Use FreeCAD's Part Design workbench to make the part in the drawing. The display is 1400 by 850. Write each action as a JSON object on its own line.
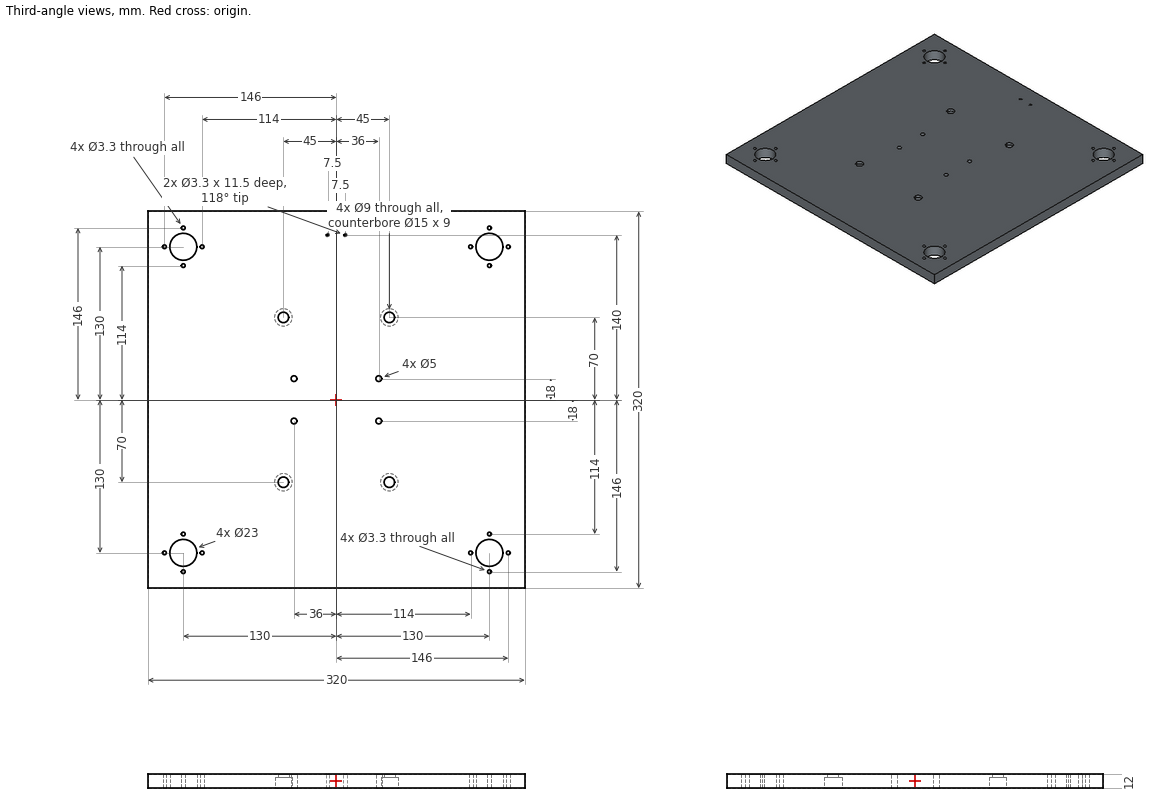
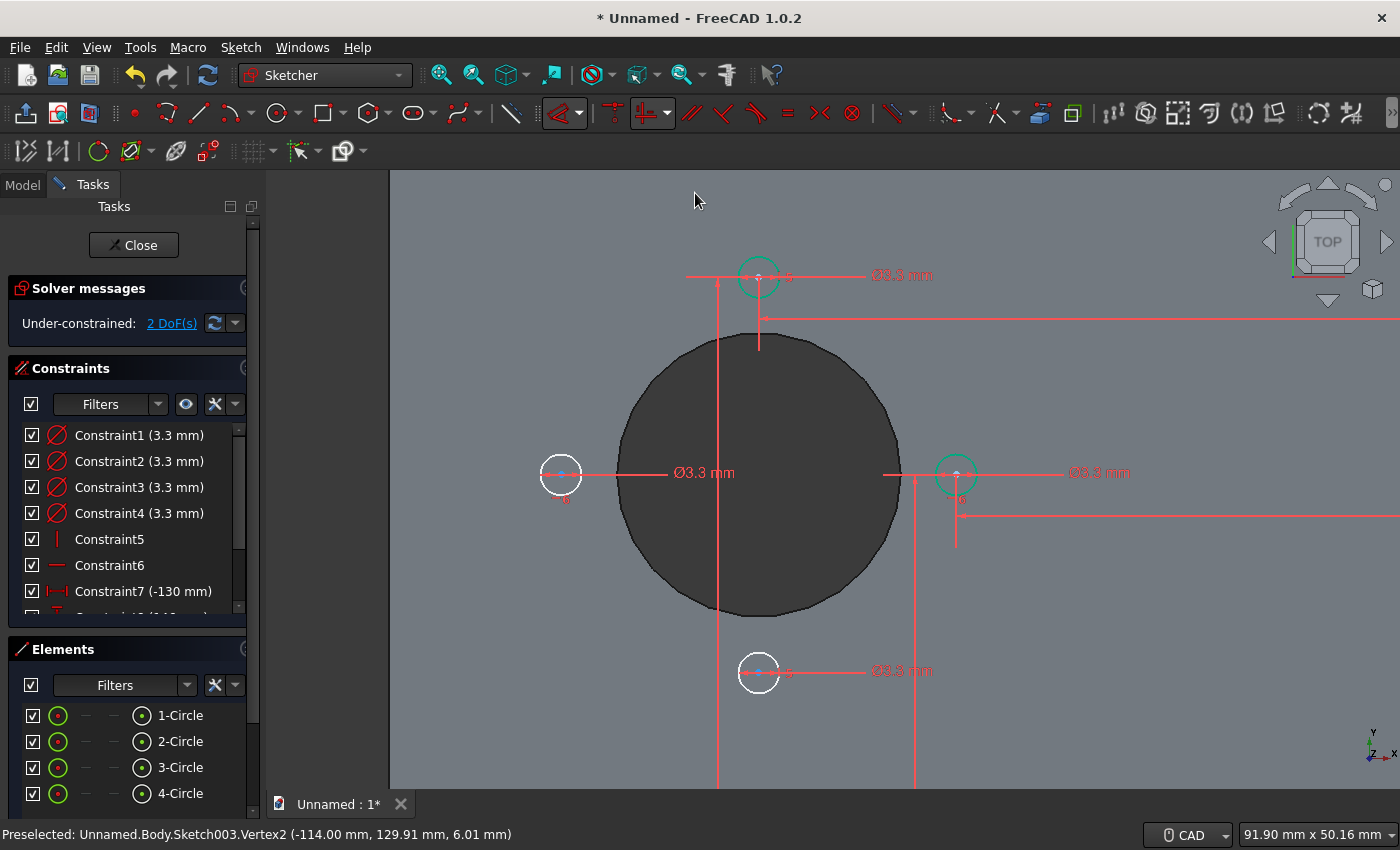
{"action": "left_click", "coordinate": [759, 673]}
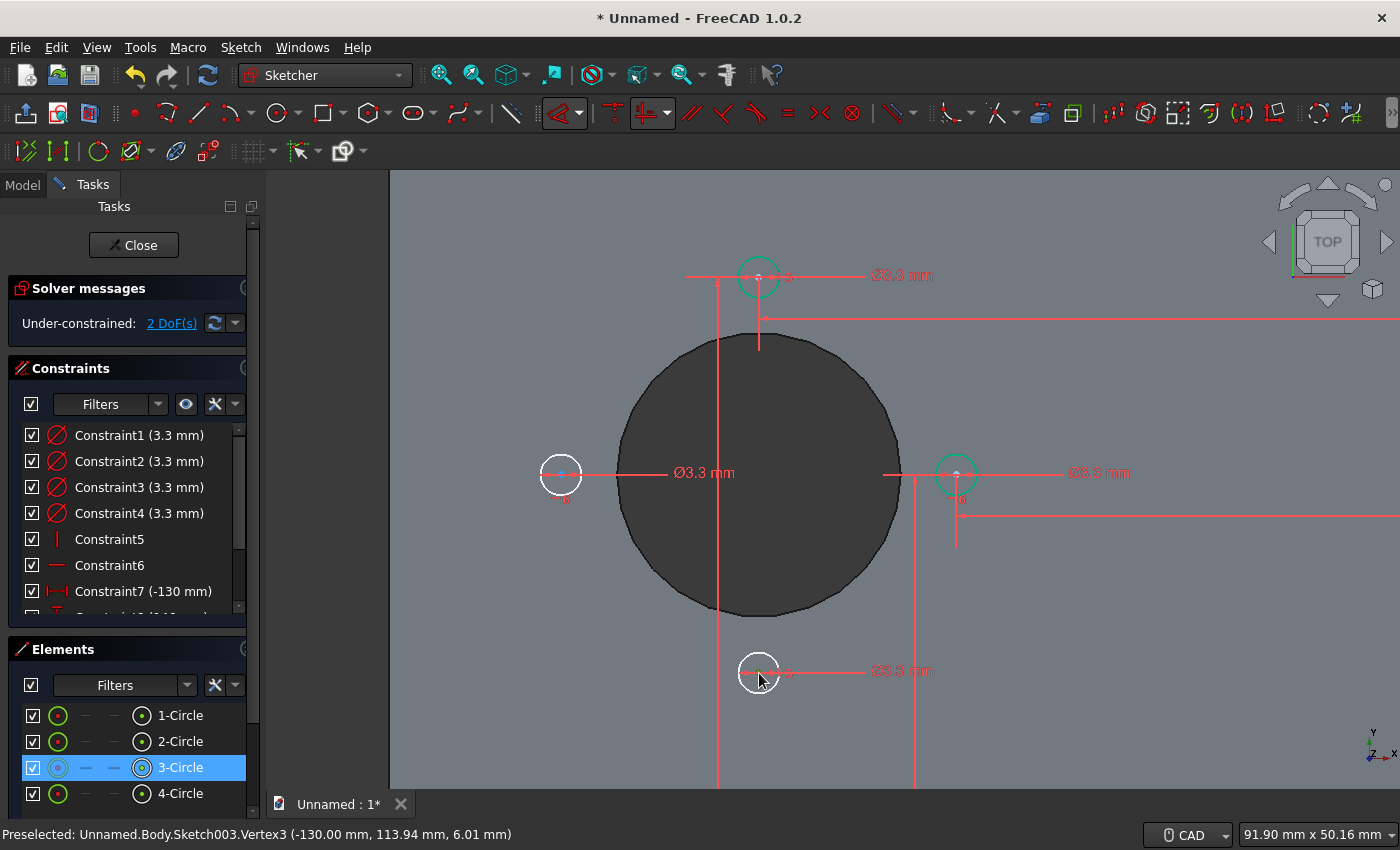
{"action": "key", "text": "i"}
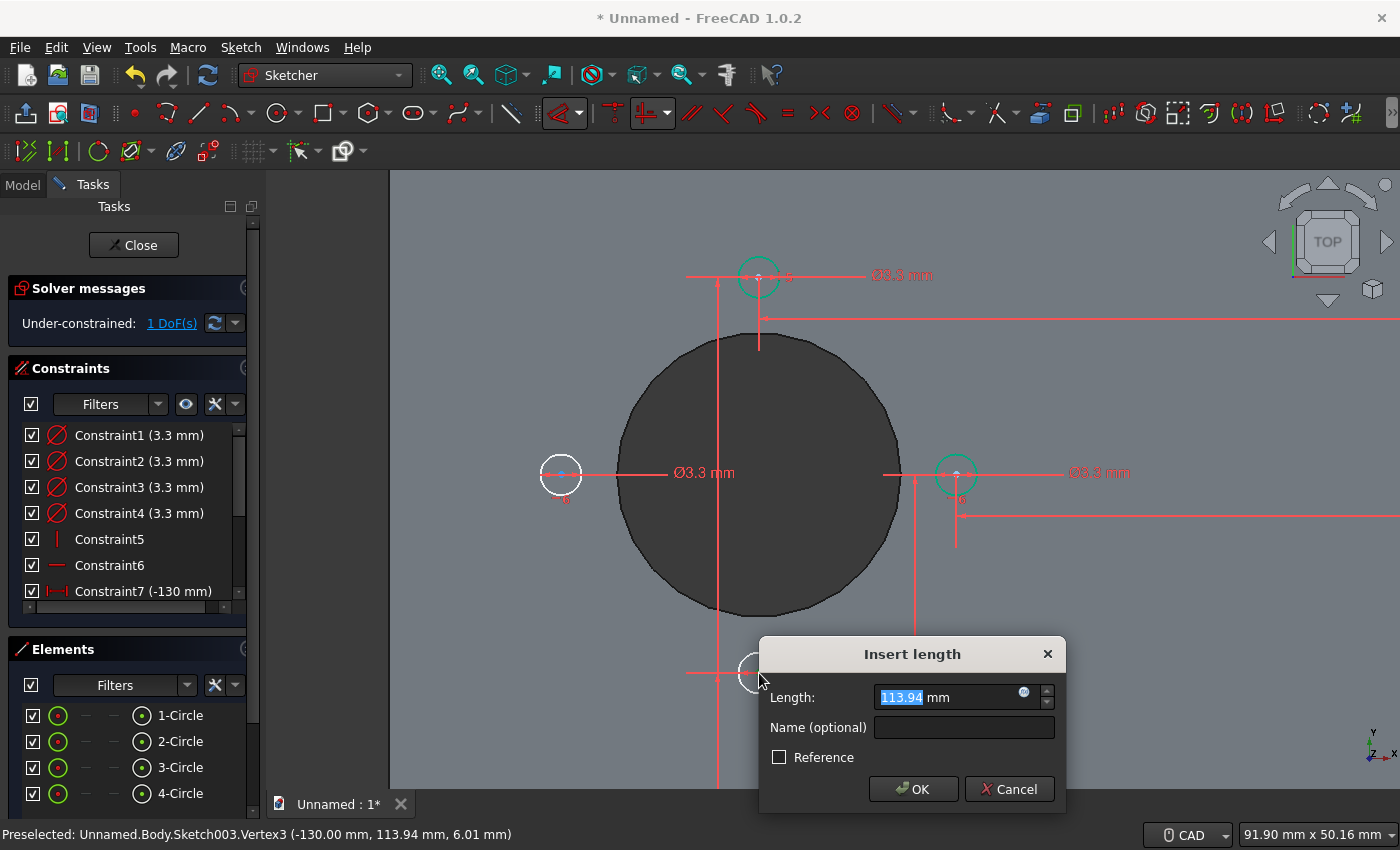
{"action": "type", "text": "114"}
{"action": "key", "text": "Return"}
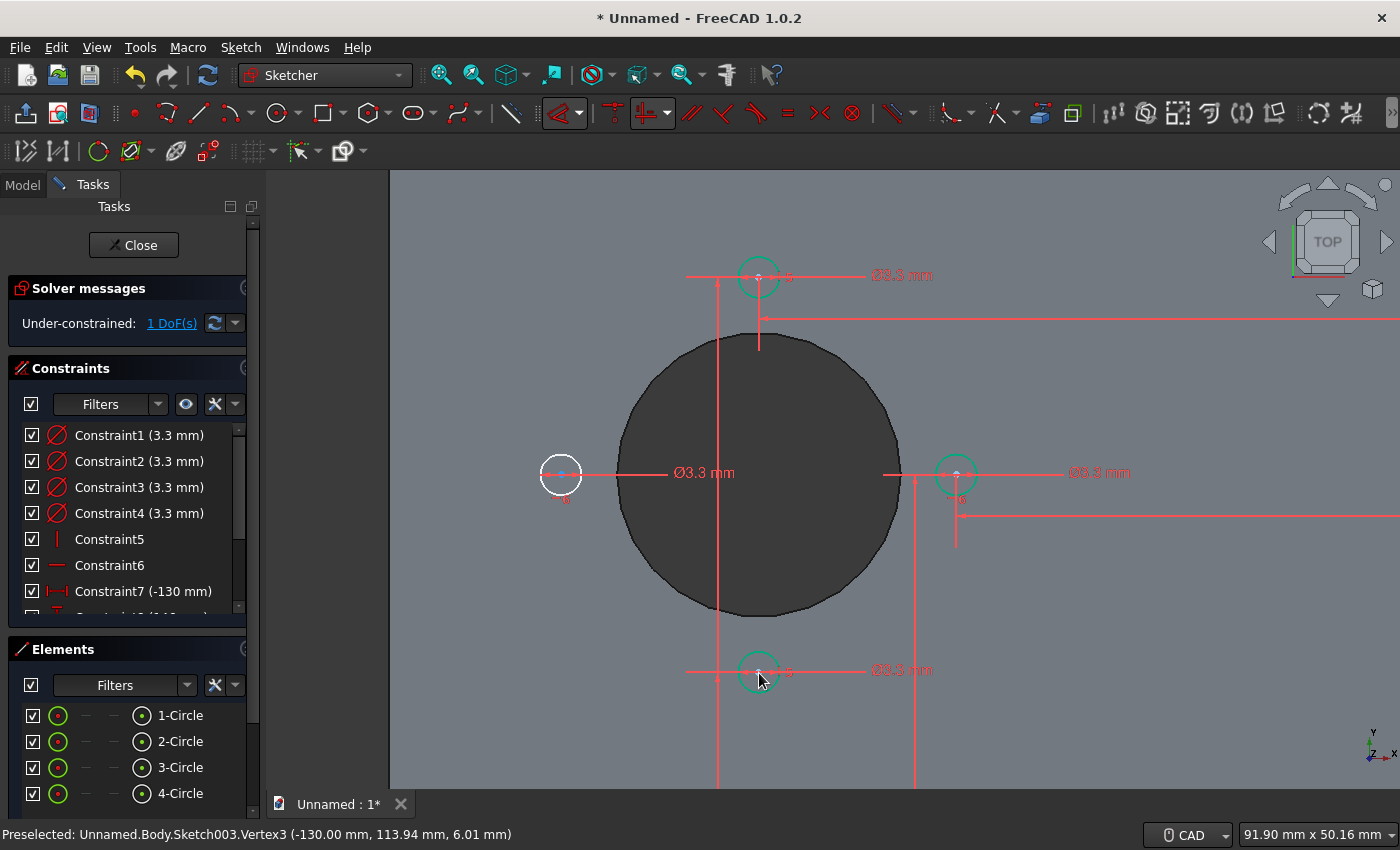
{"action": "left_click", "coordinate": [561, 475]}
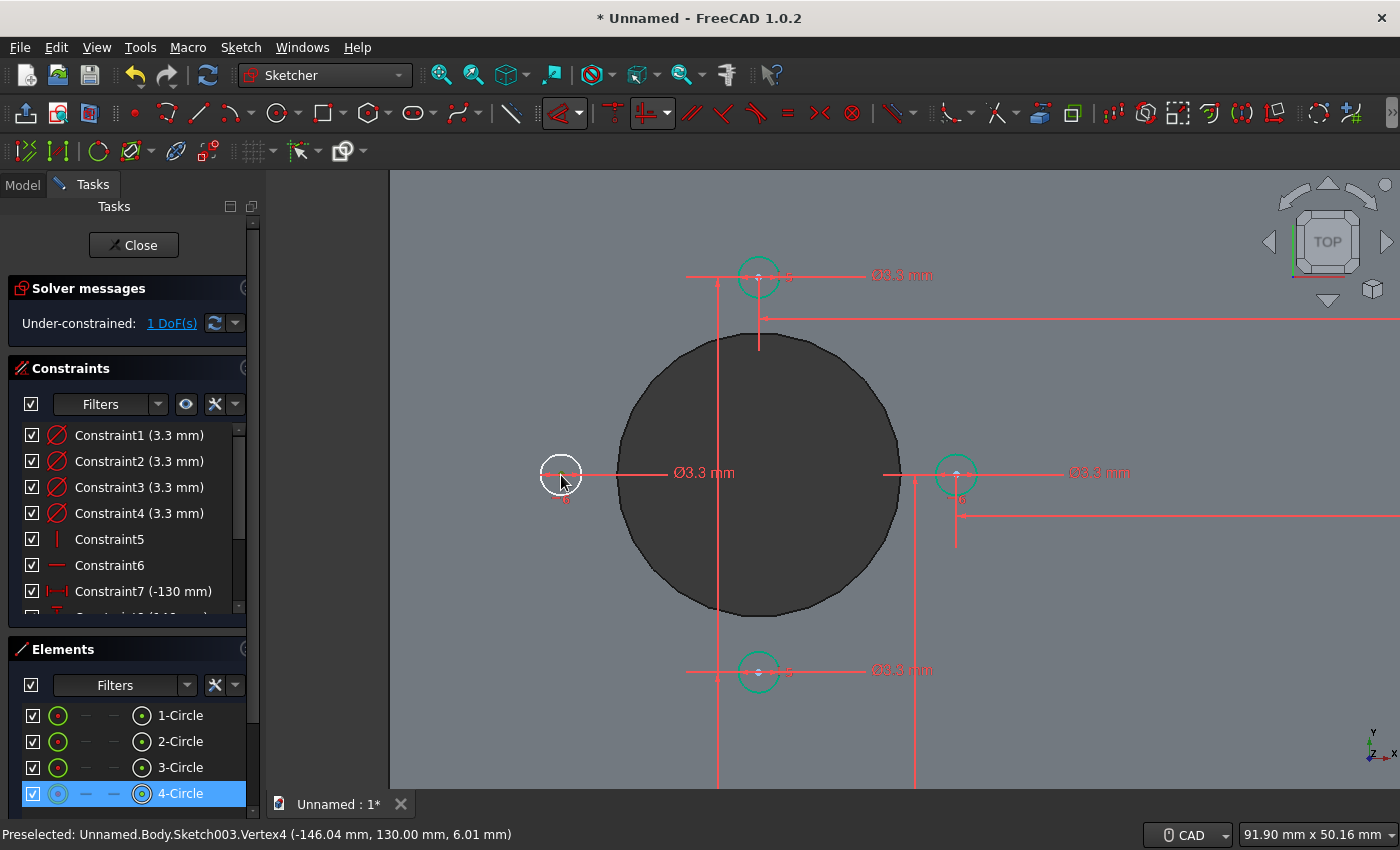
{"action": "left_click", "coordinate": [582, 114]}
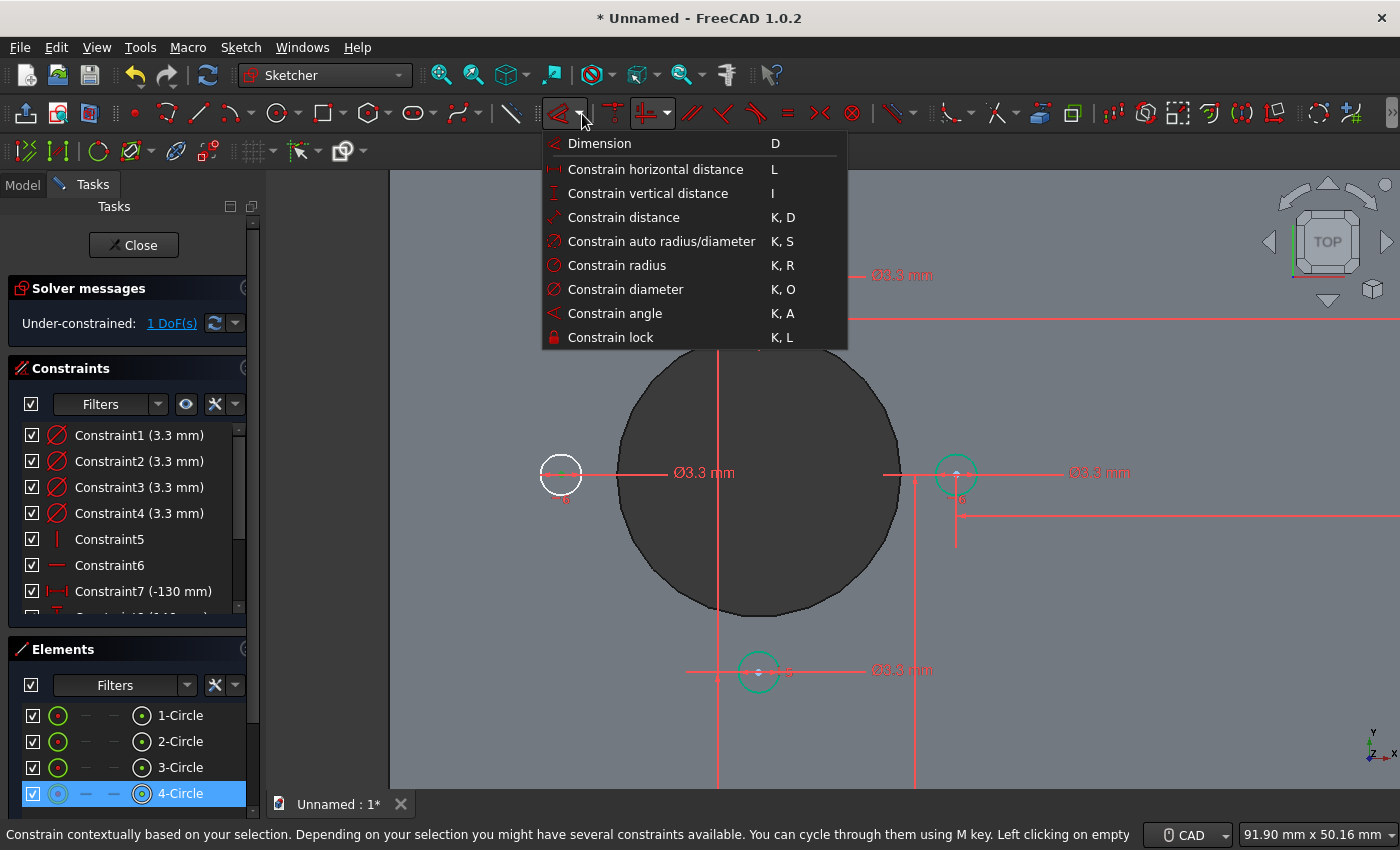
{"action": "left_click", "coordinate": [695, 169]}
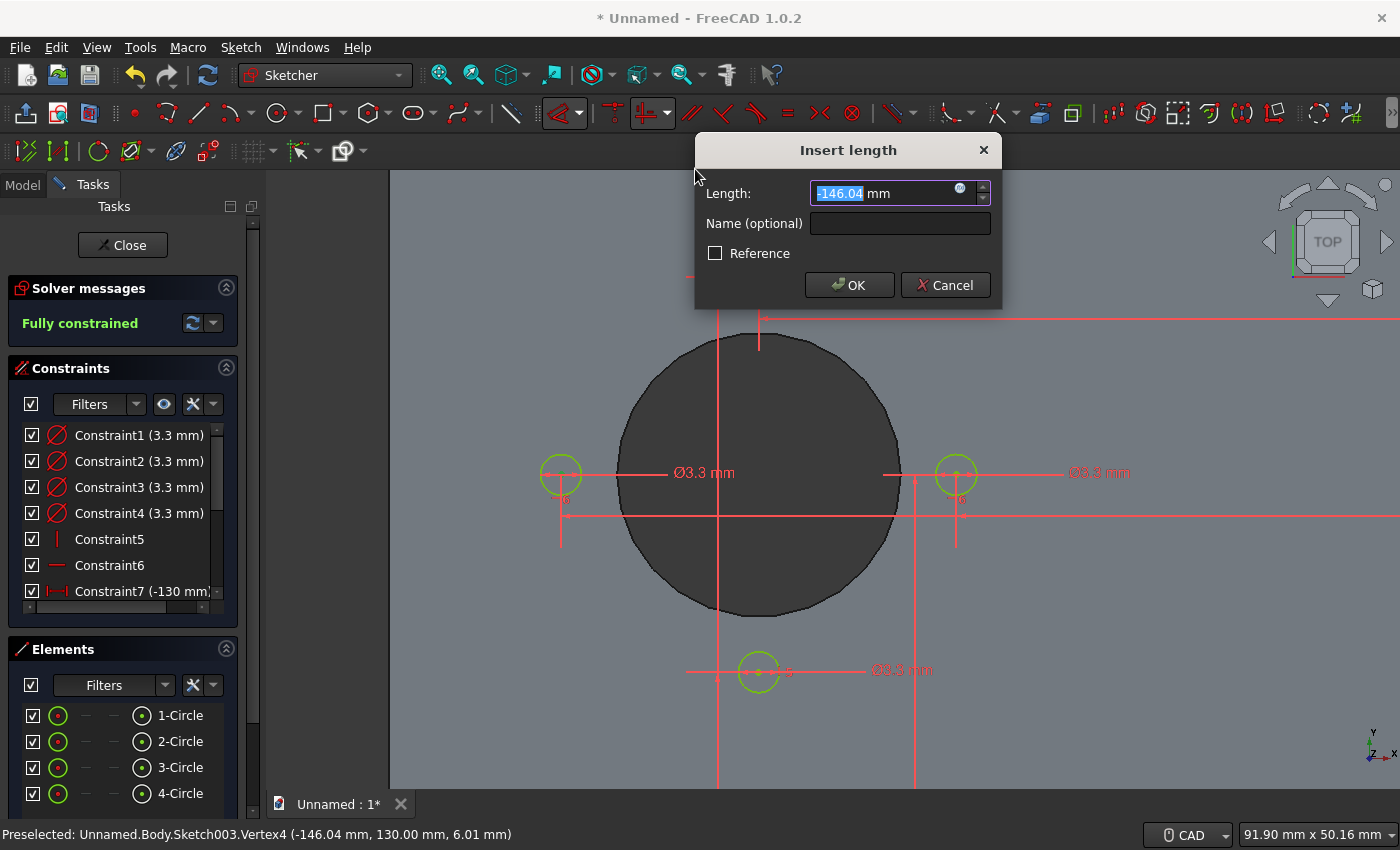
{"action": "type", "text": "-146"}
{"action": "key", "text": "Return"}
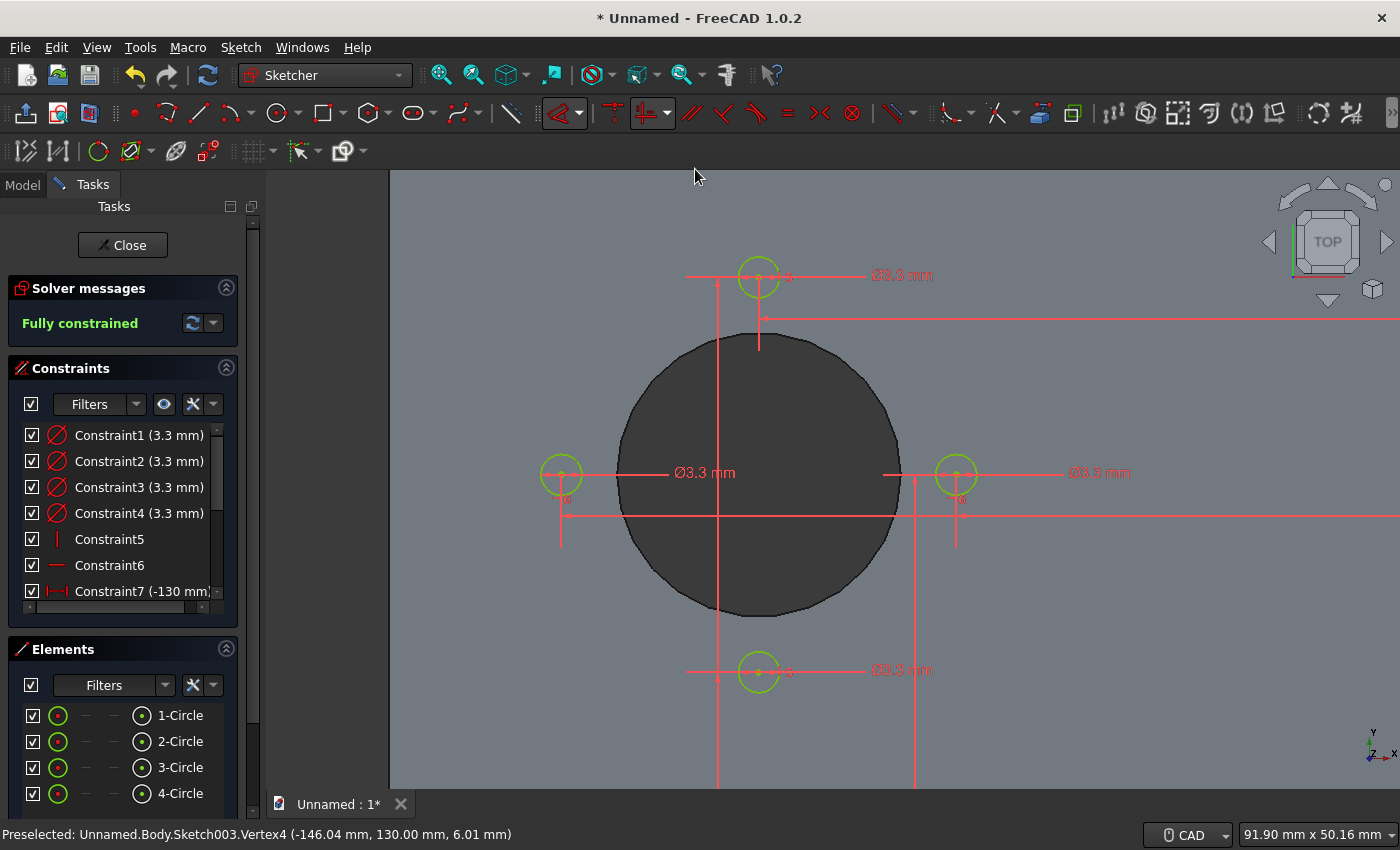
{"action": "left_click", "coordinate": [123, 245]}